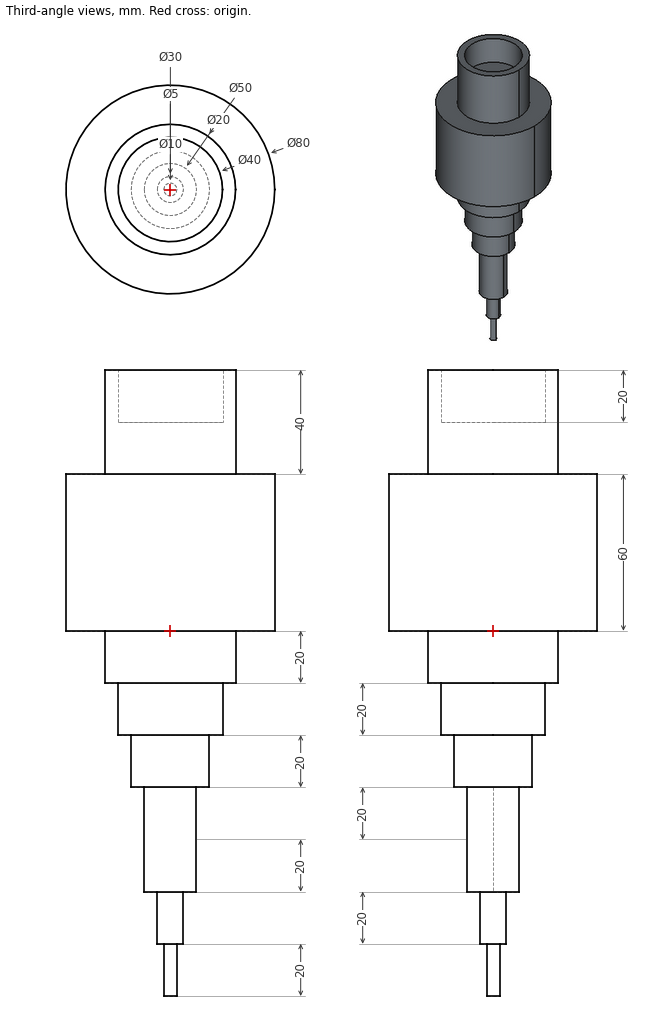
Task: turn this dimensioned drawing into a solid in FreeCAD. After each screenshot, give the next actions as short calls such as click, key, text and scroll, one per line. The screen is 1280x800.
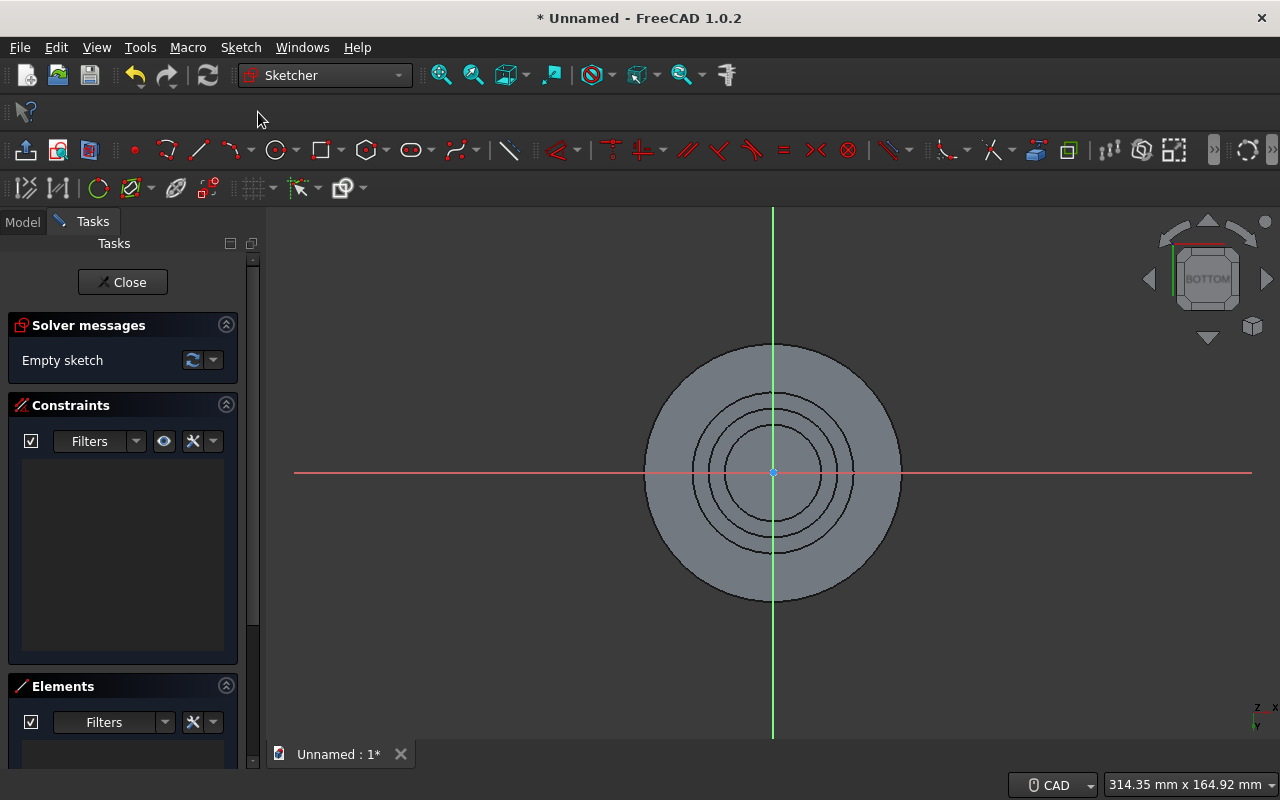
scroll(790, 473, up, 8)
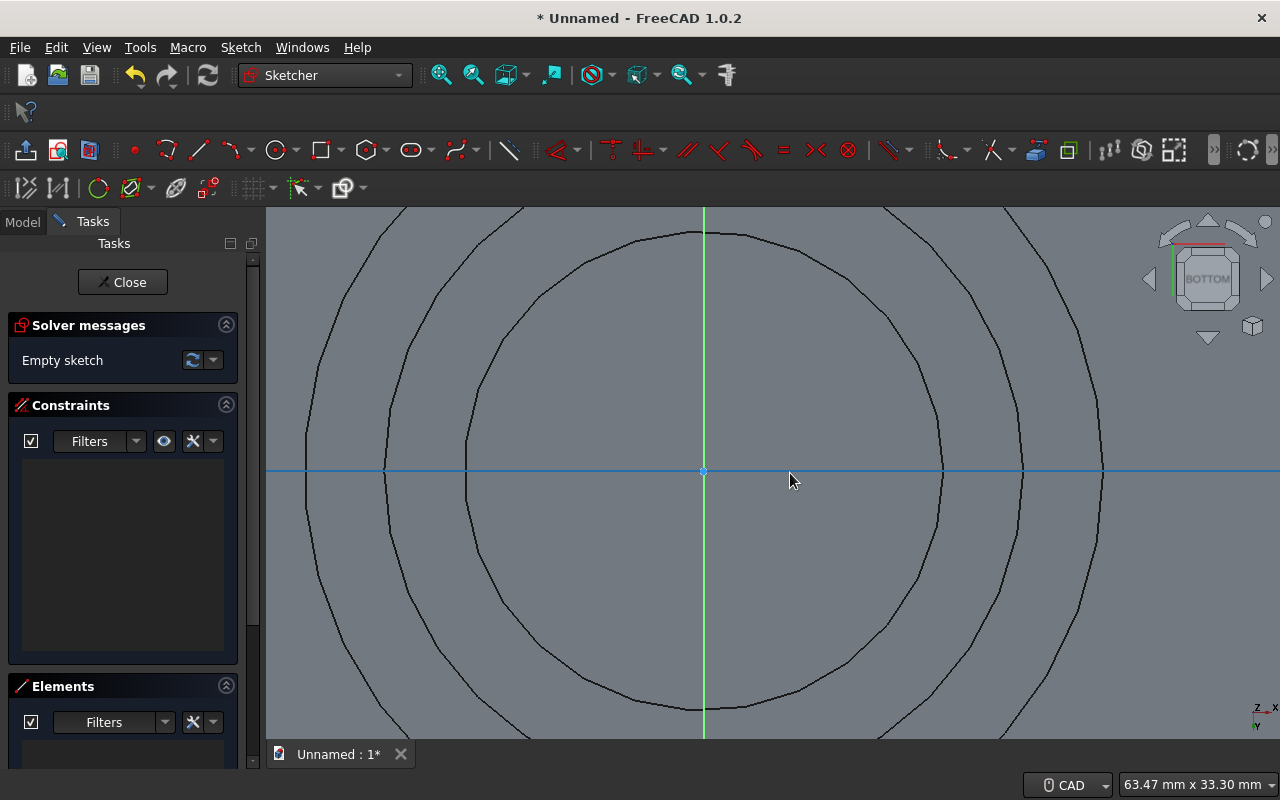
click(276, 150)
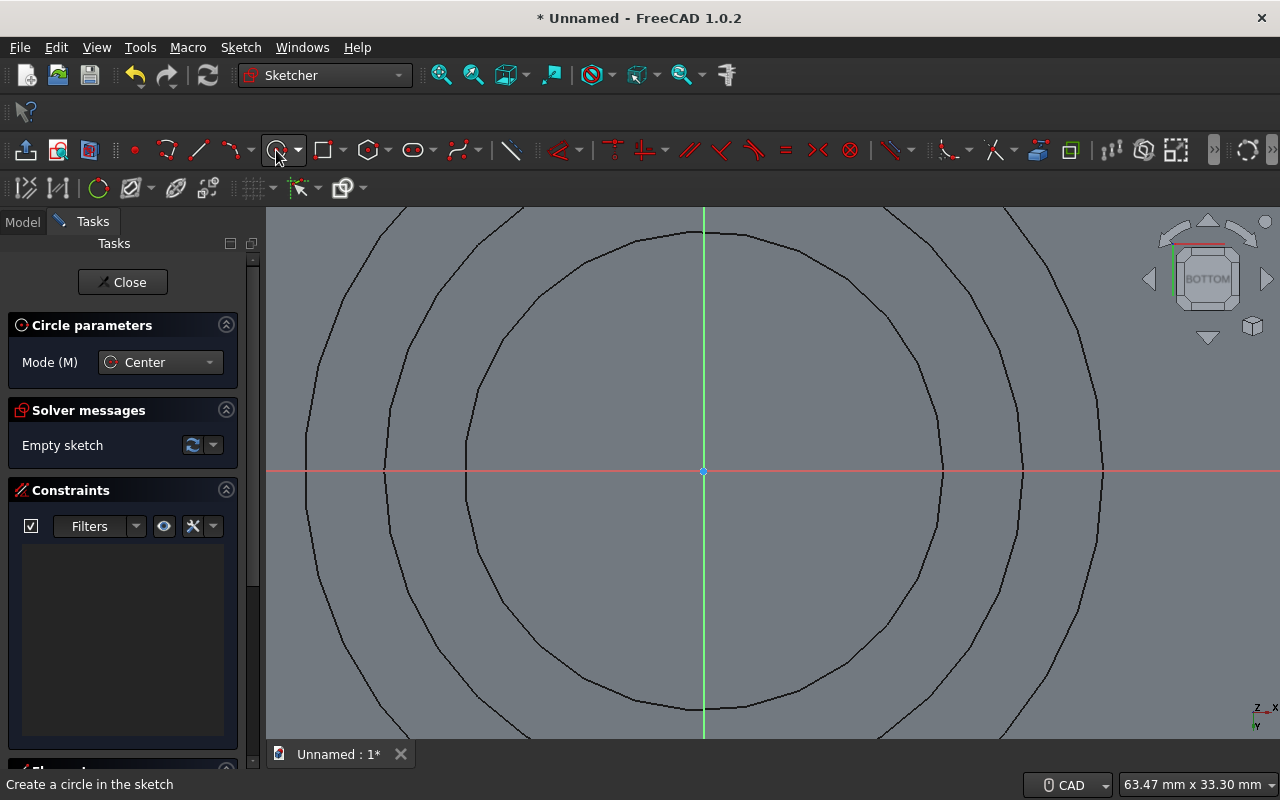
click(704, 471)
click(817, 358)
key(Escape)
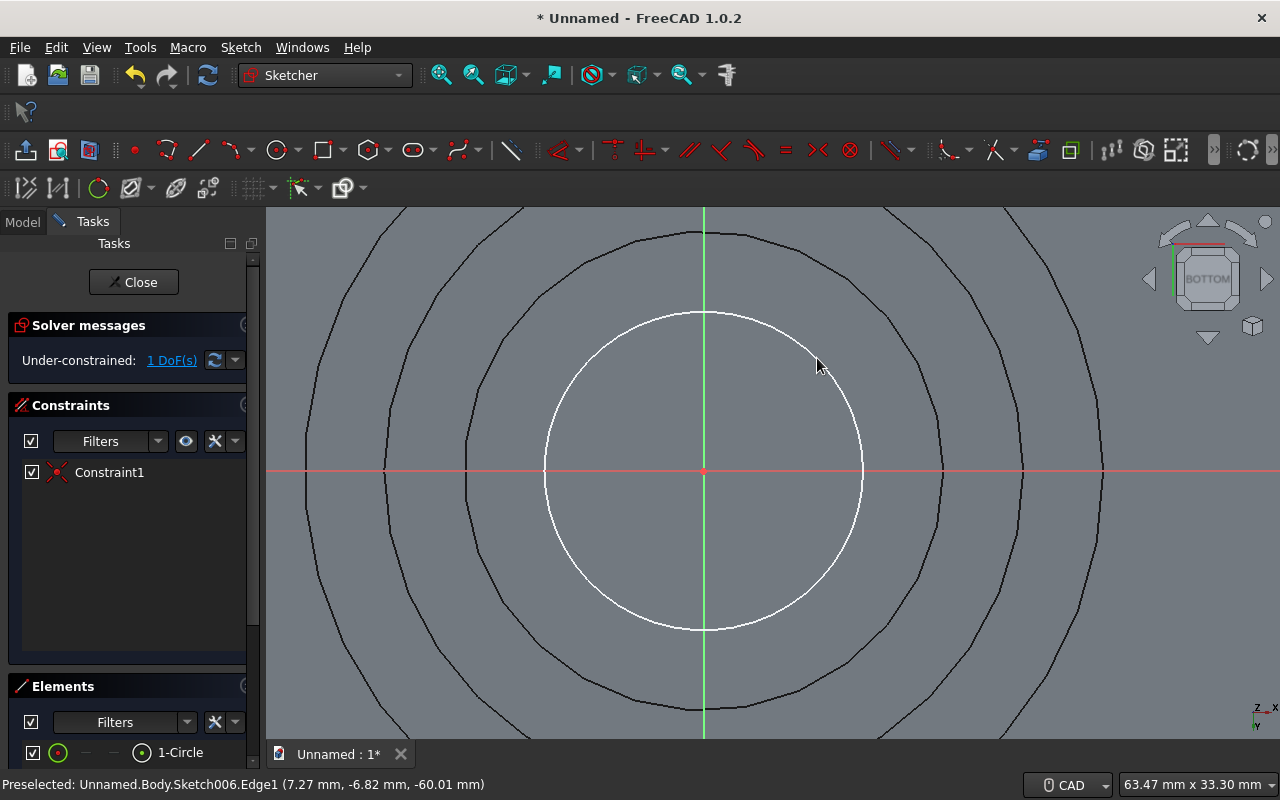
click(558, 150)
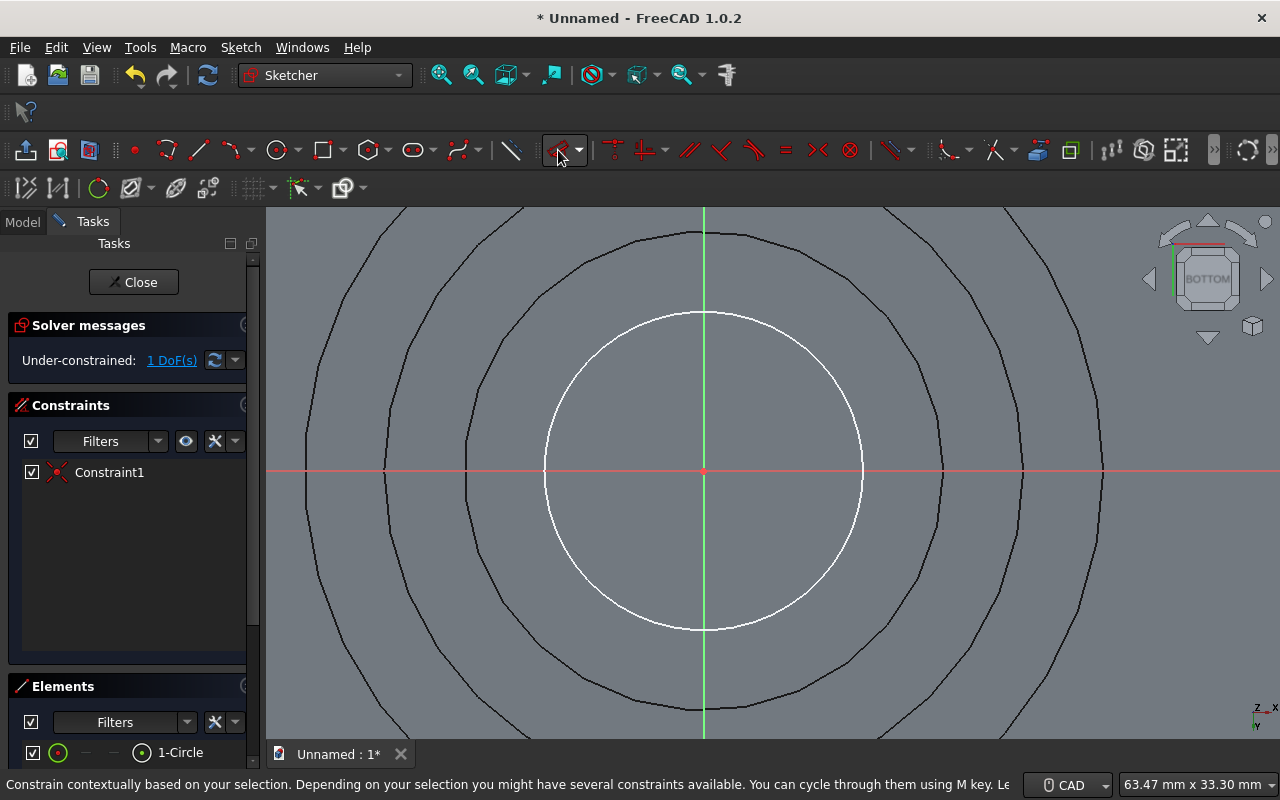
click(816, 358)
click(839, 335)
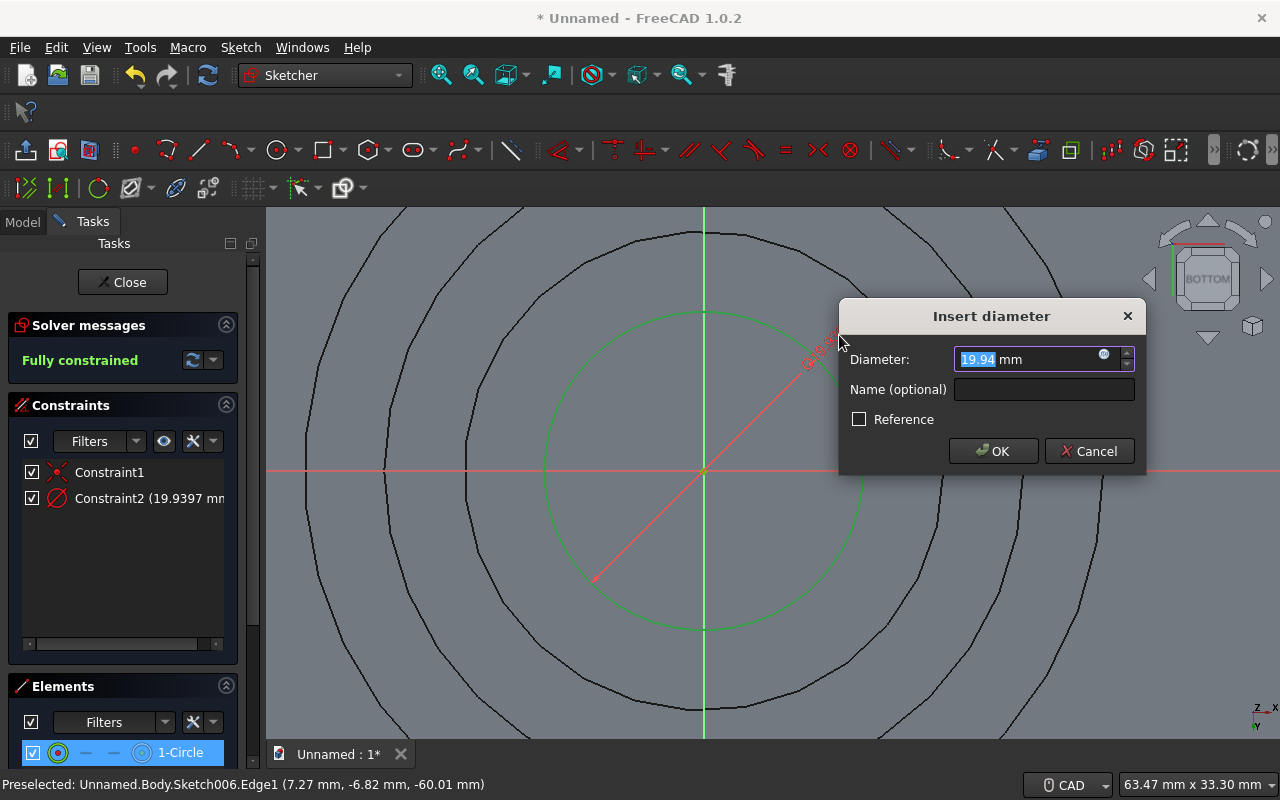
text(20)
key(Return)
key(Escape)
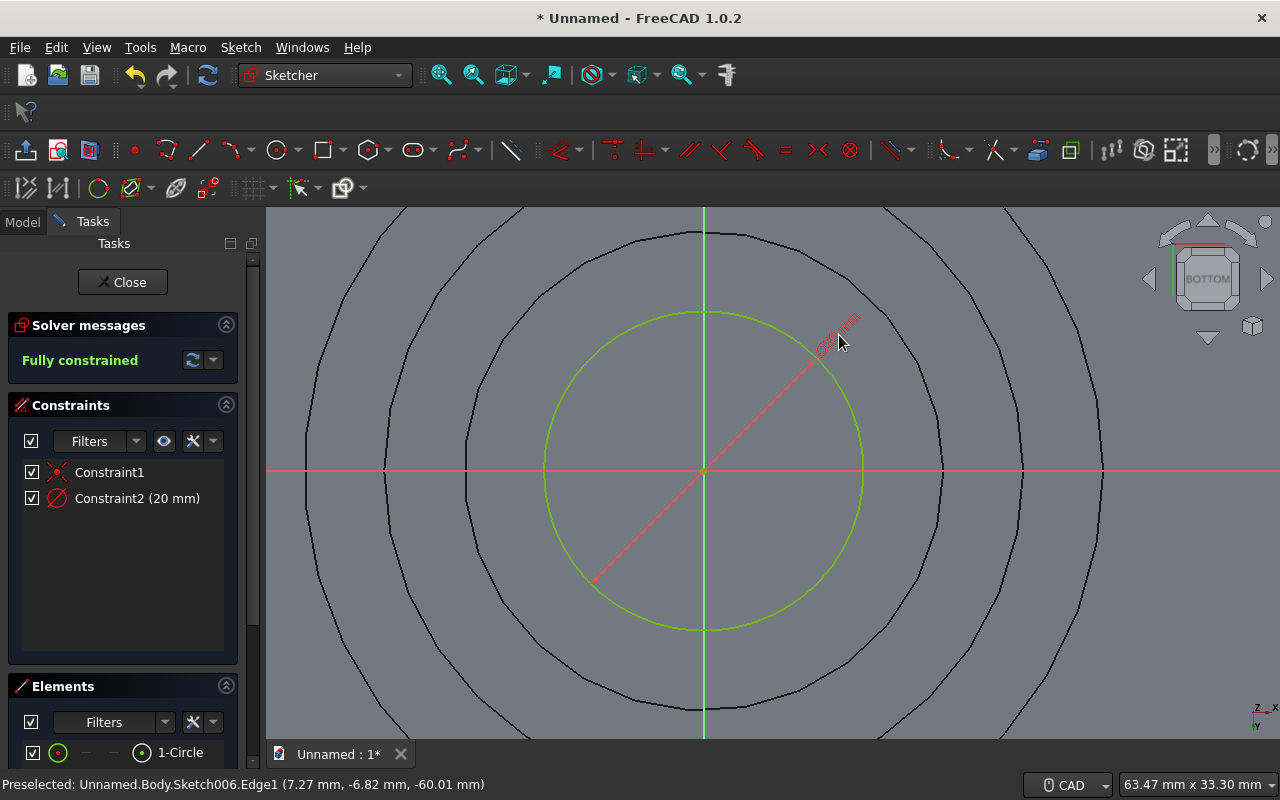
click(123, 282)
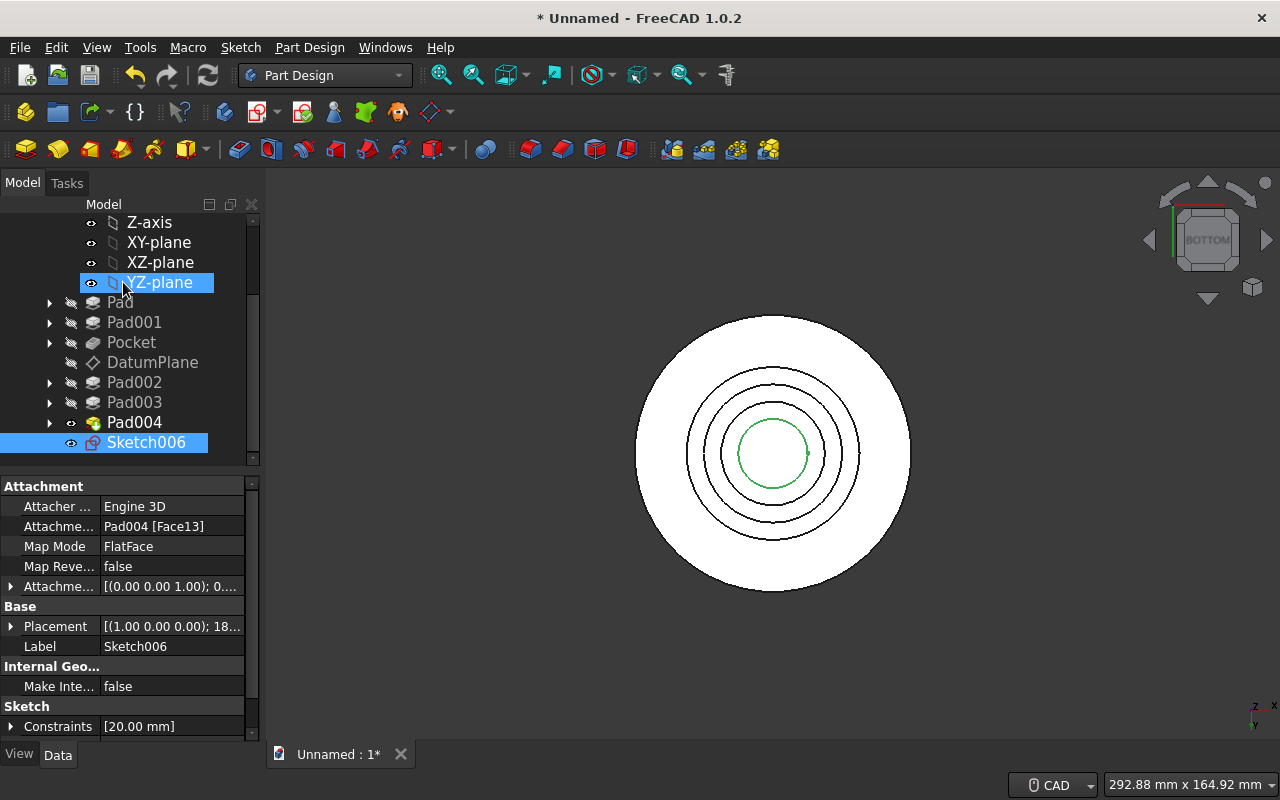
click(26, 150)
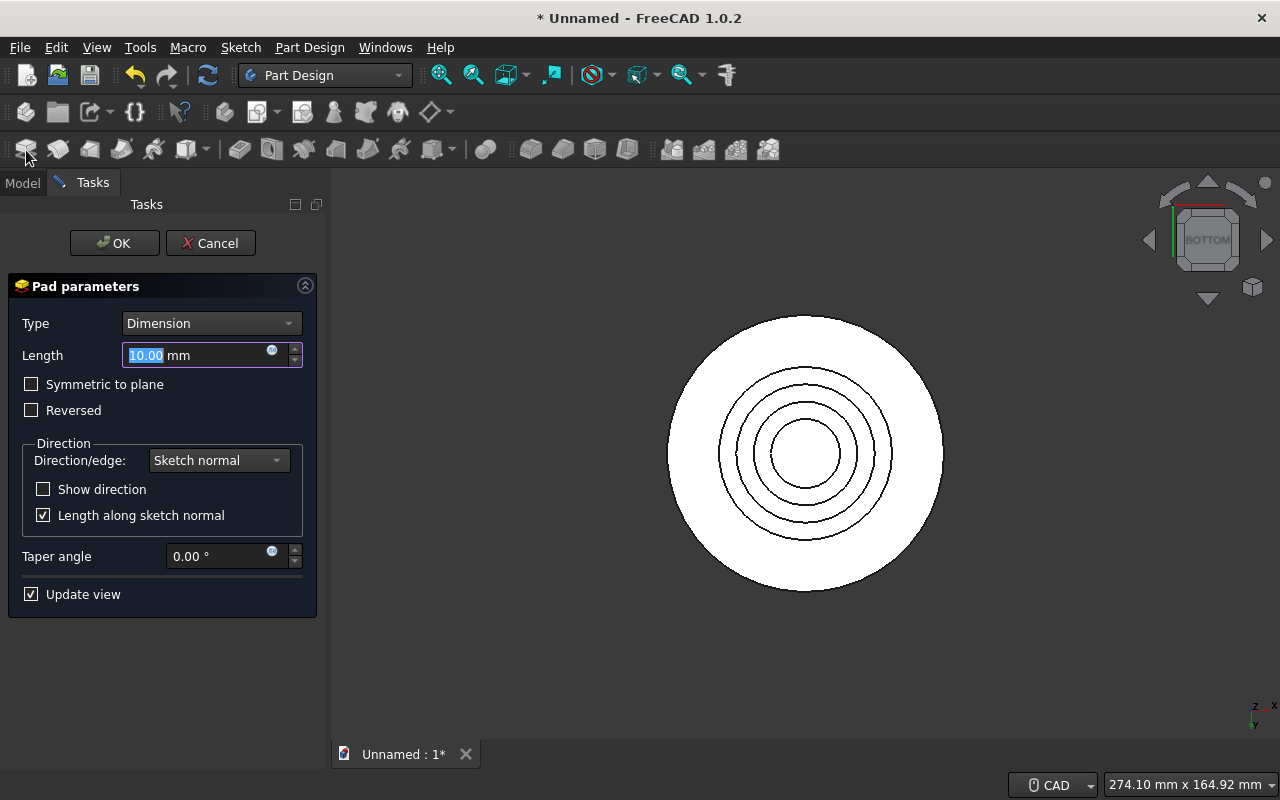
text(20)
key(Tab)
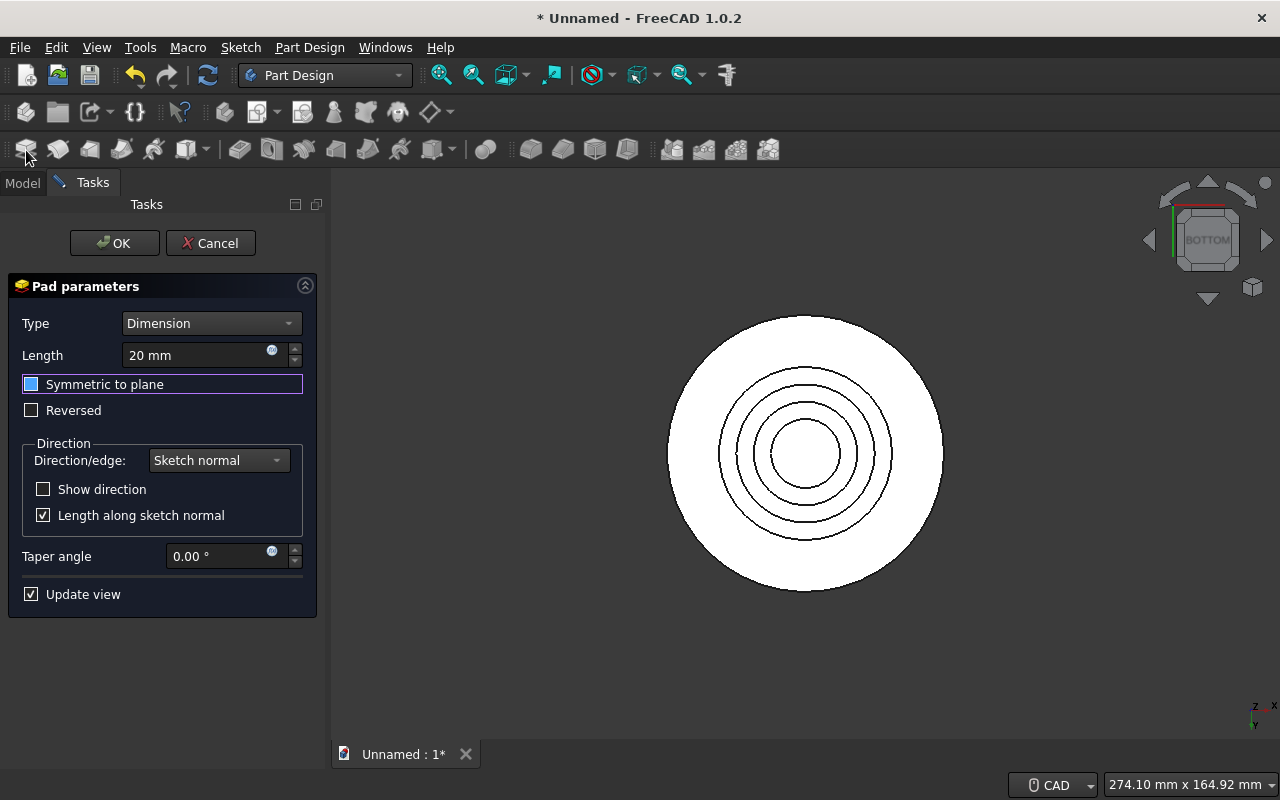
click(115, 243)